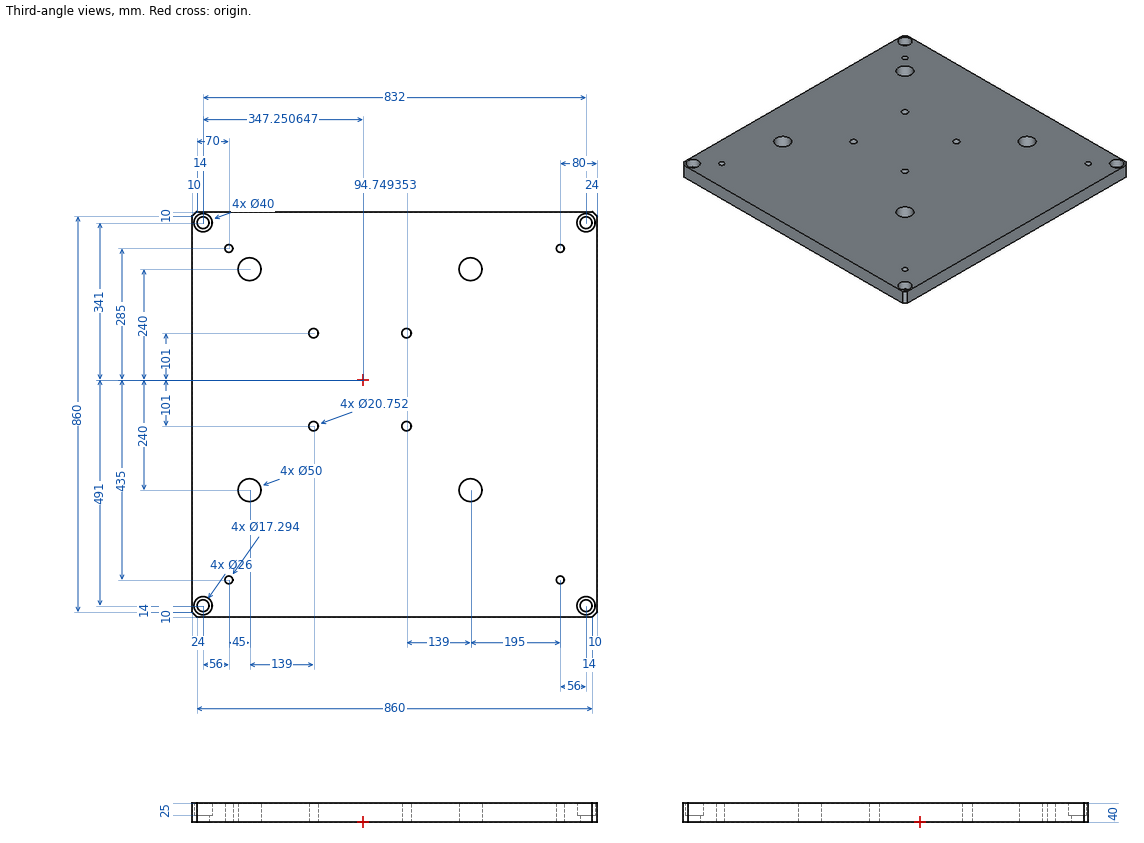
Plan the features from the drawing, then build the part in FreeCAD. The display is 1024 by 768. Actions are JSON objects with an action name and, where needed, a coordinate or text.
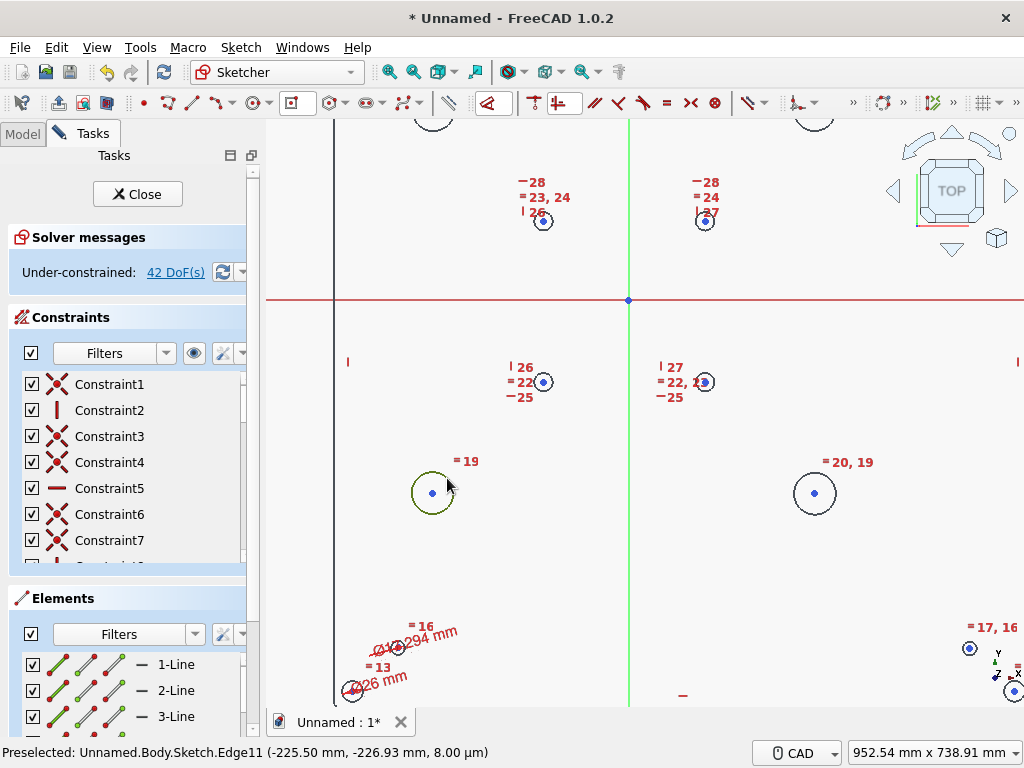
{"action": "left_click", "coordinate": [506, 104]}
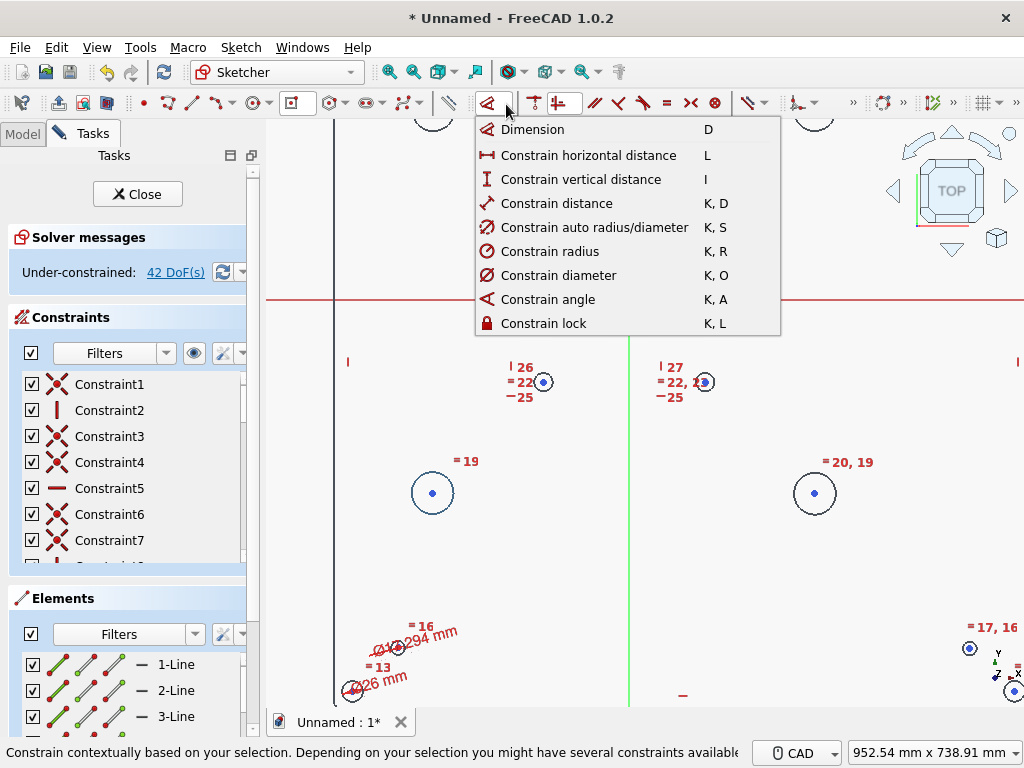
{"action": "left_click", "coordinate": [628, 275]}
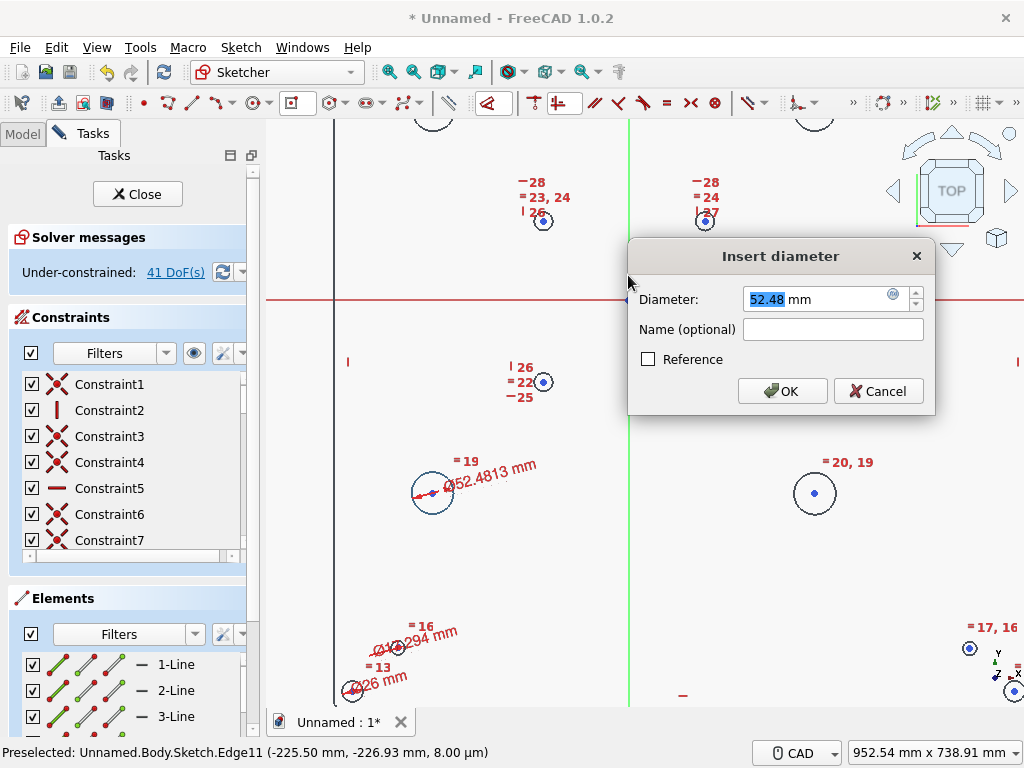
{"action": "type", "text": "50"}
{"action": "key", "text": "Return"}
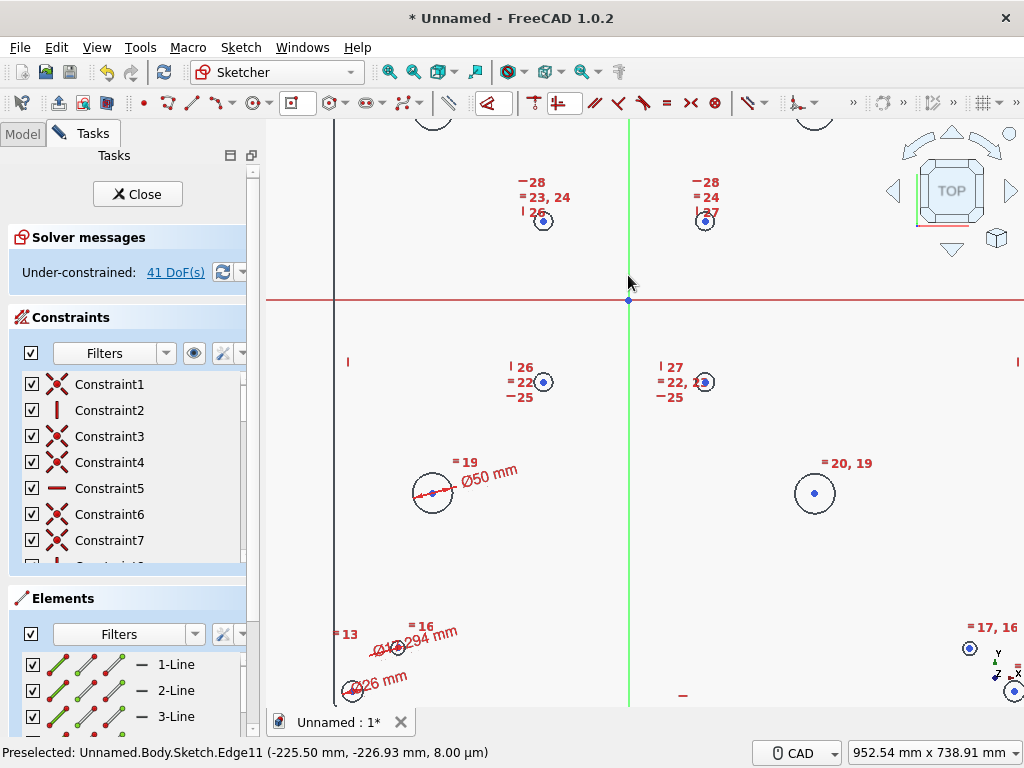
{"action": "scroll", "coordinate": [550, 376], "scroll_direction": "up", "scroll_amount": 5}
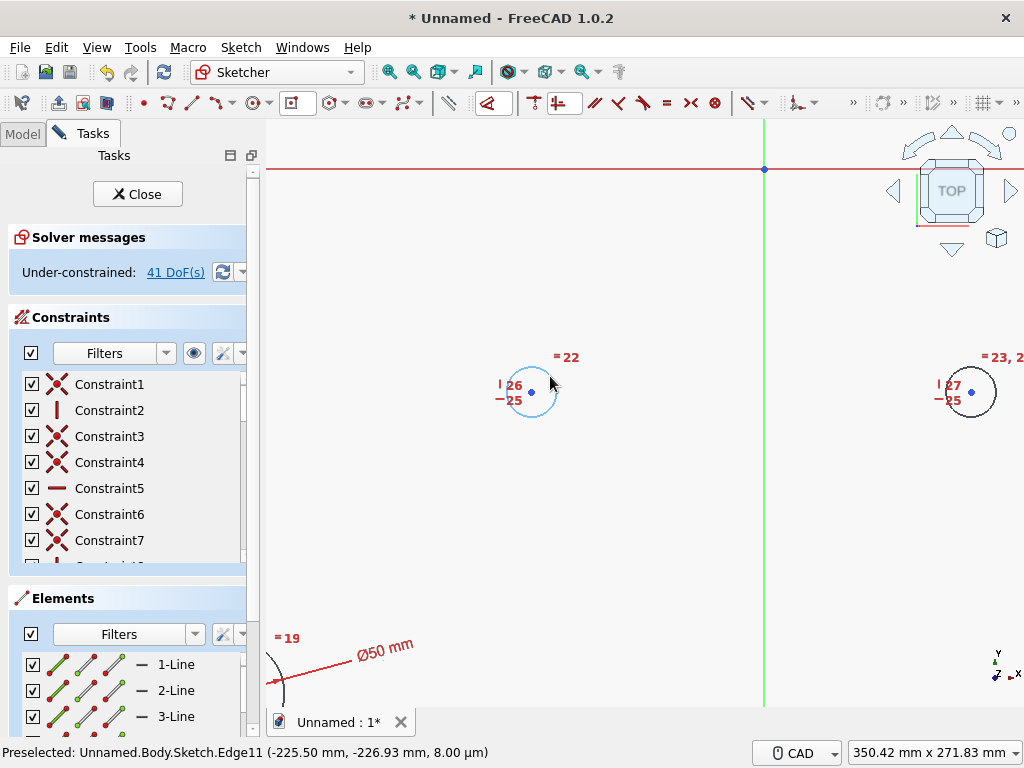
{"action": "left_click", "coordinate": [549, 374]}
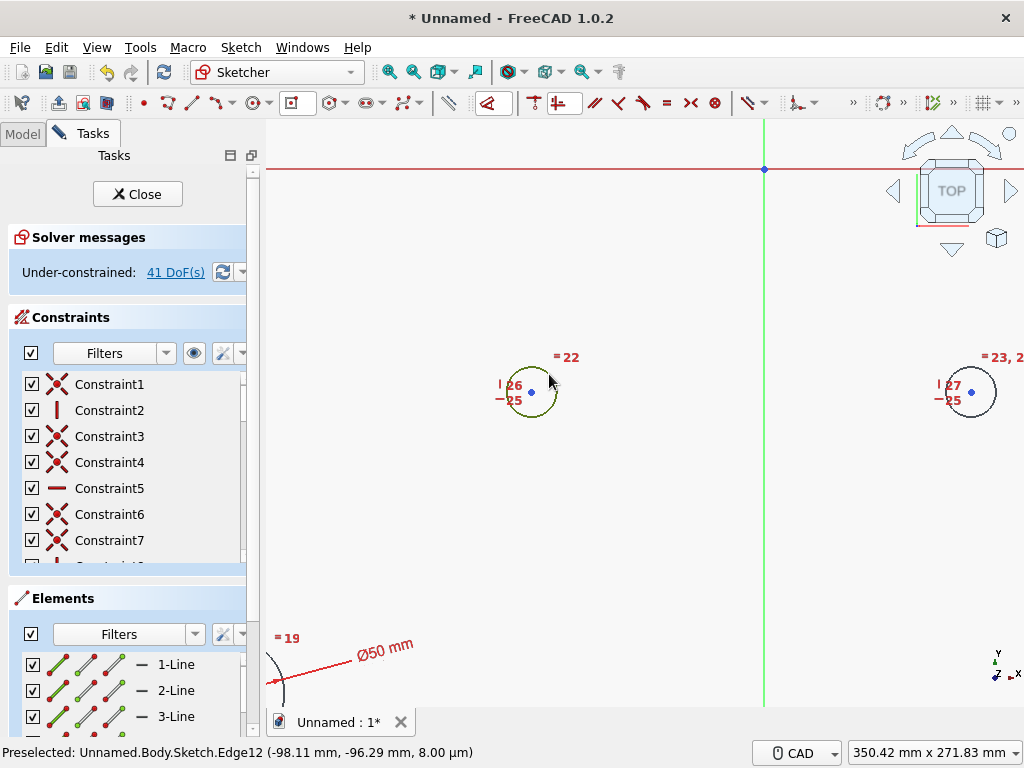
{"action": "left_click", "coordinate": [506, 104]}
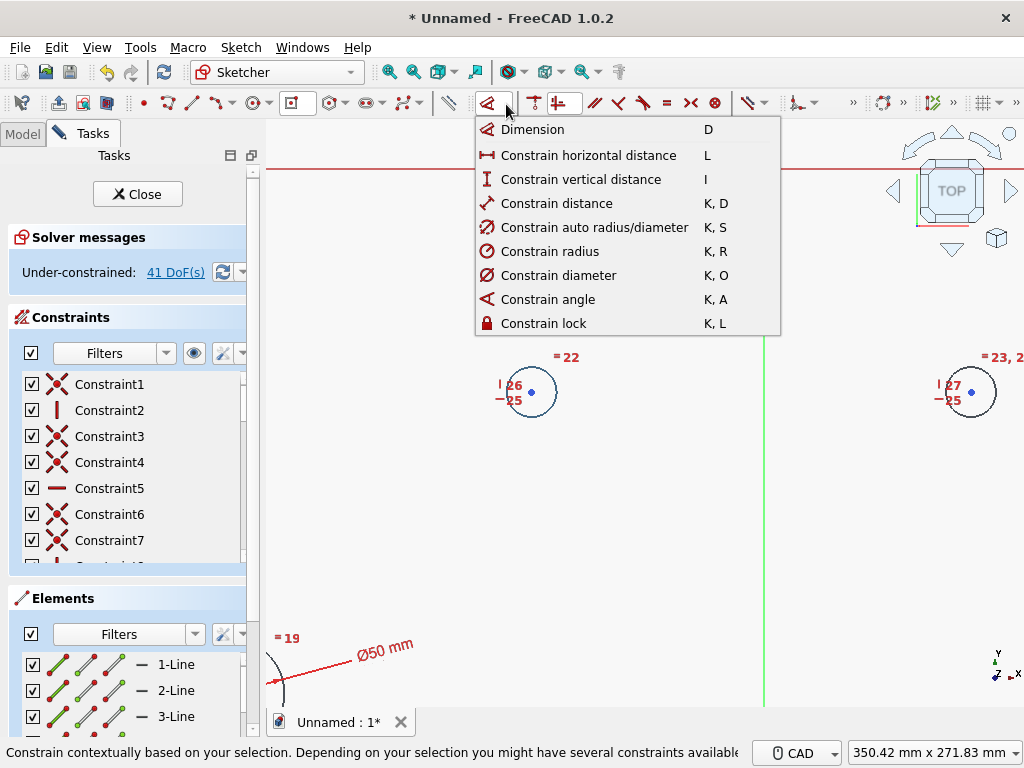
{"action": "left_click", "coordinate": [628, 275]}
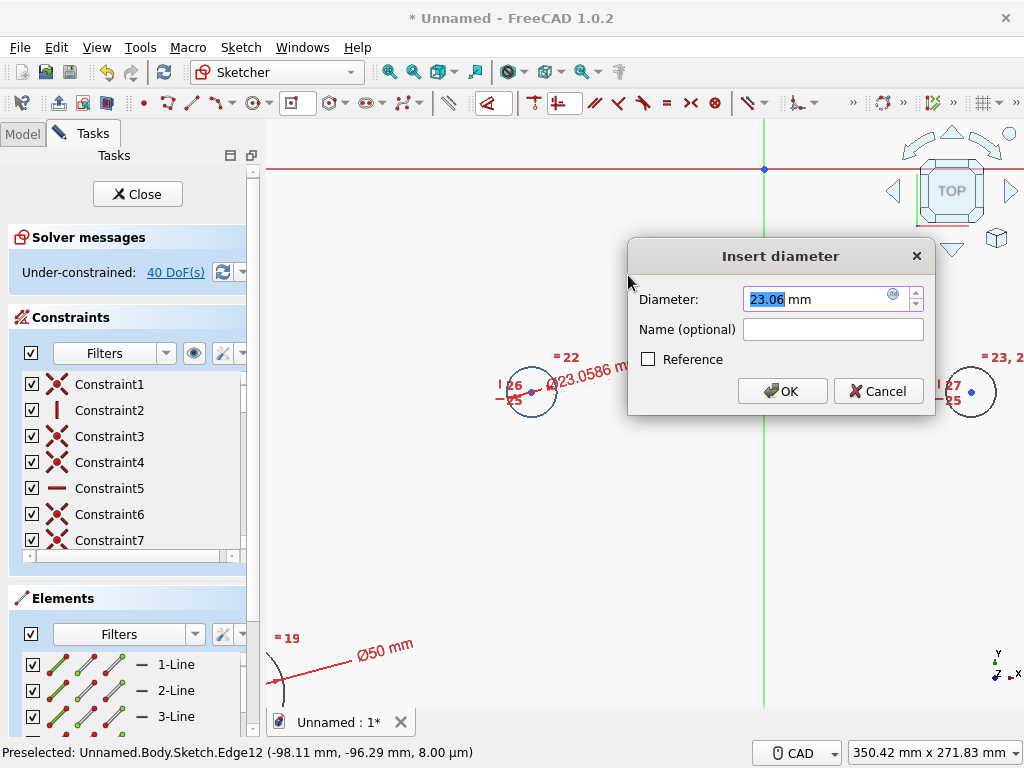
{"action": "type", "text": "20.752"}
{"action": "key", "text": "Return"}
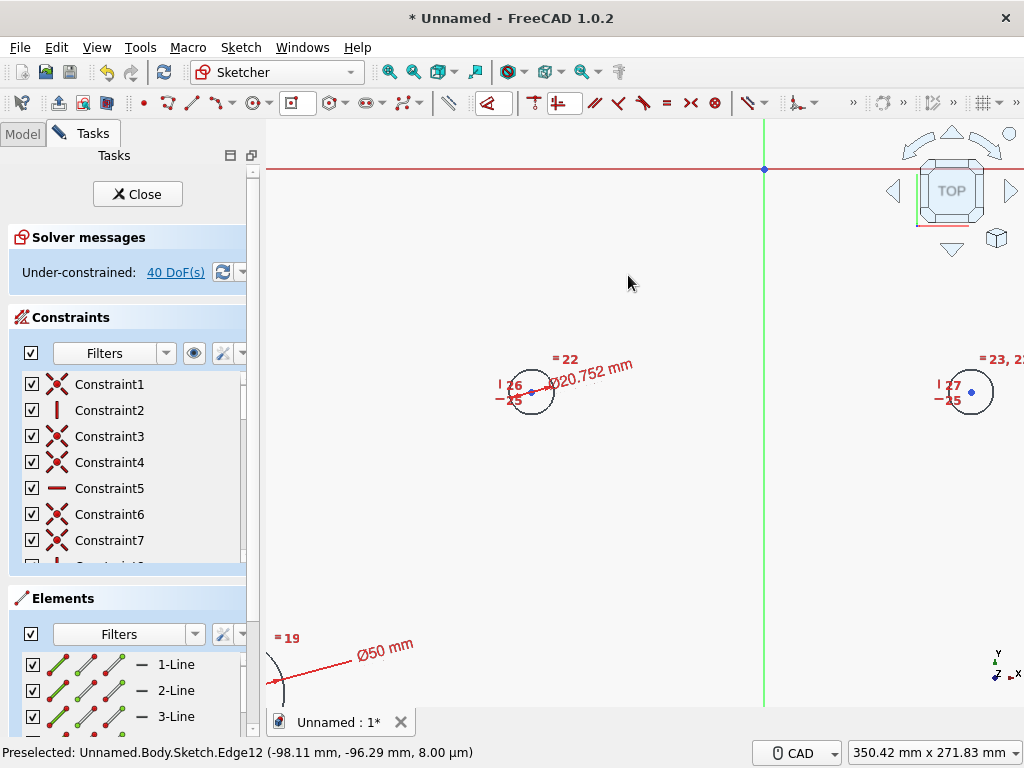
{"action": "scroll", "coordinate": [491, 434], "scroll_direction": "down", "scroll_amount": 8}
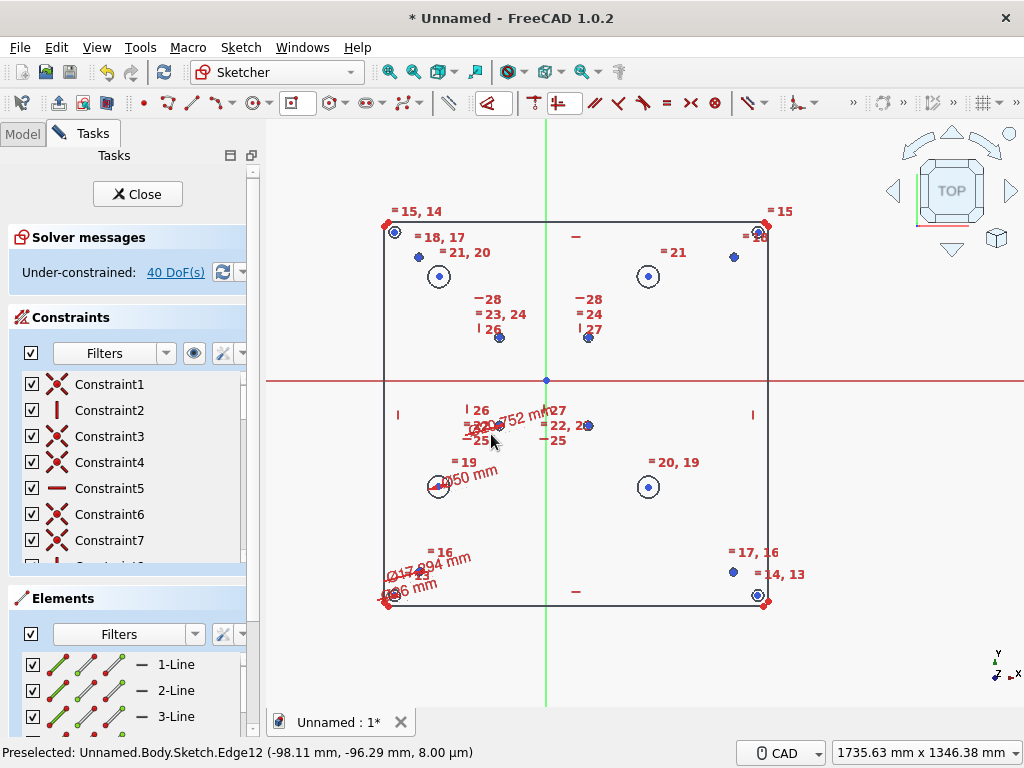
{"action": "left_click", "coordinate": [384, 339]}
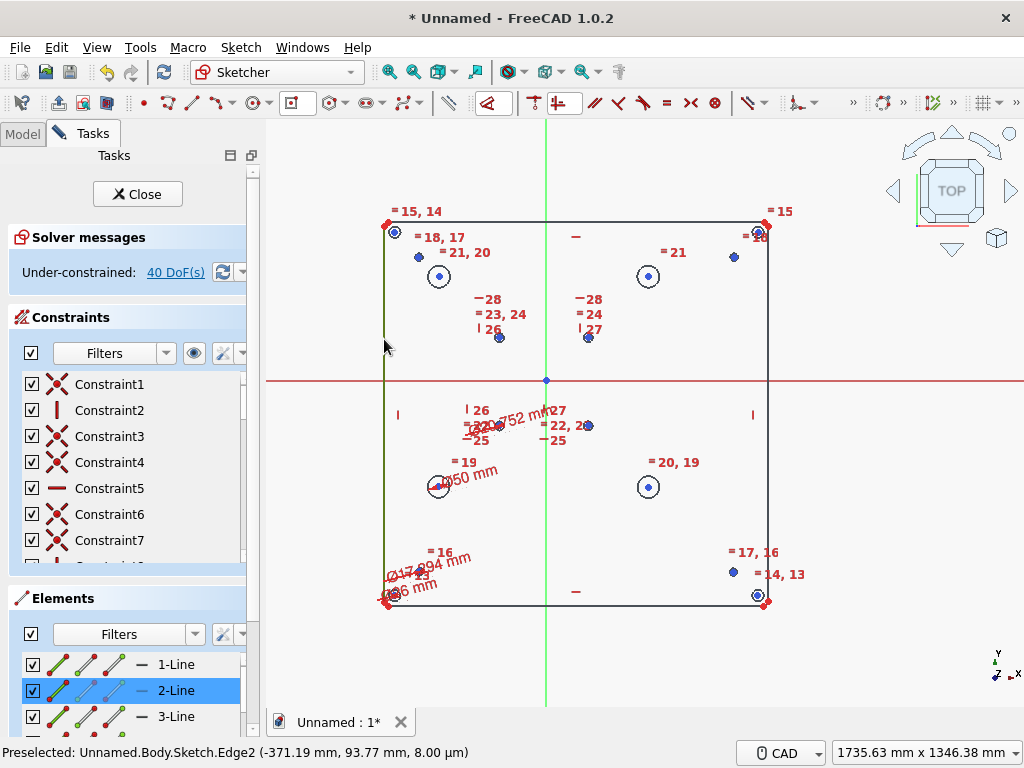
{"action": "key", "text": "i"}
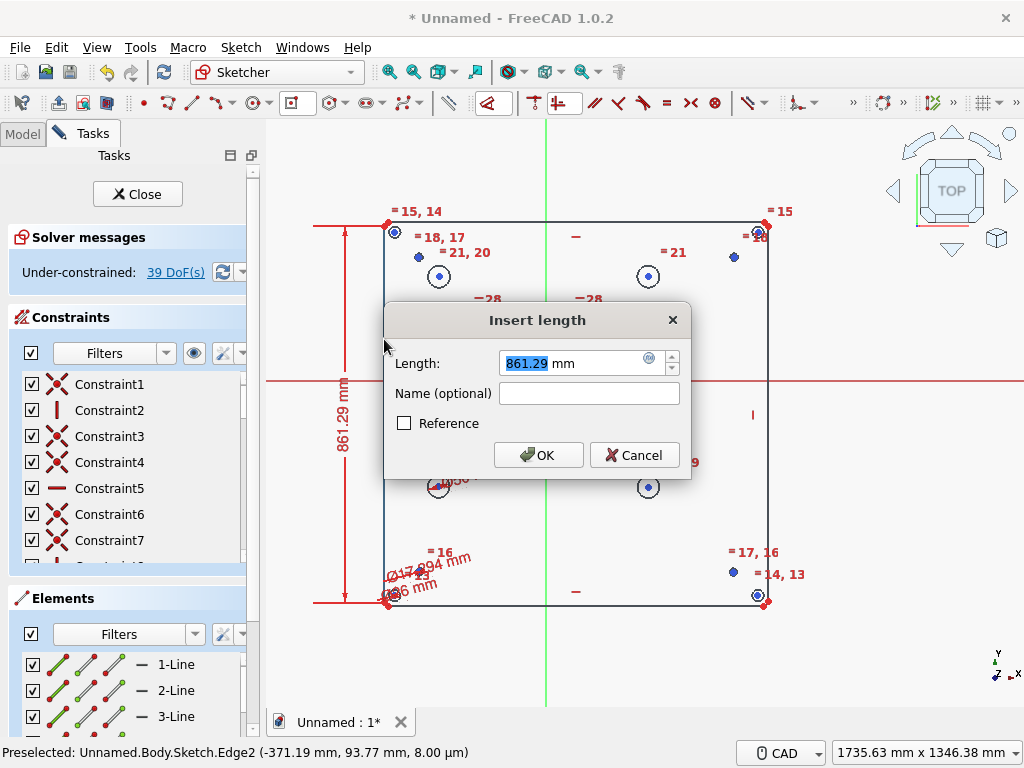
{"action": "type", "text": "860"}
{"action": "key", "text": "Return"}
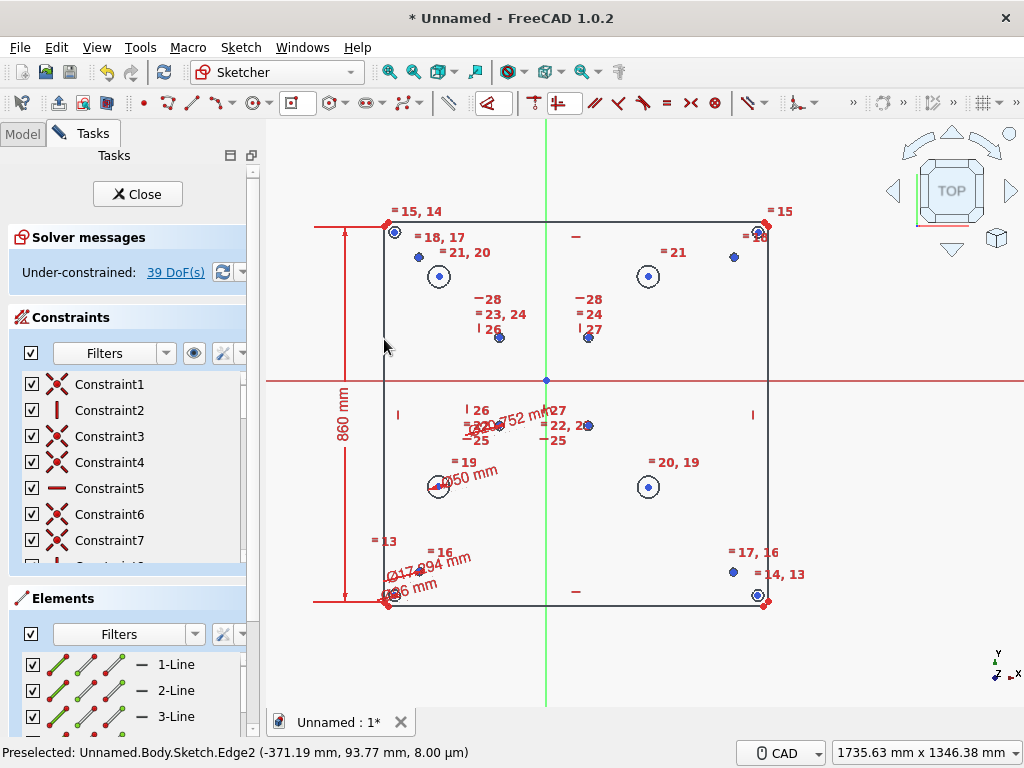
{"action": "left_click", "coordinate": [501, 606]}